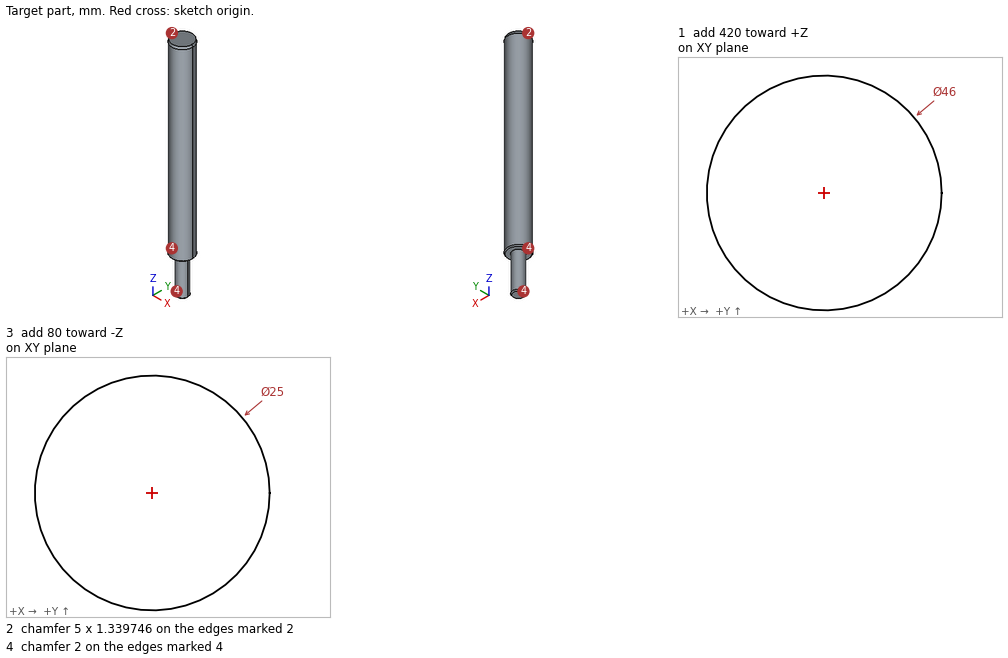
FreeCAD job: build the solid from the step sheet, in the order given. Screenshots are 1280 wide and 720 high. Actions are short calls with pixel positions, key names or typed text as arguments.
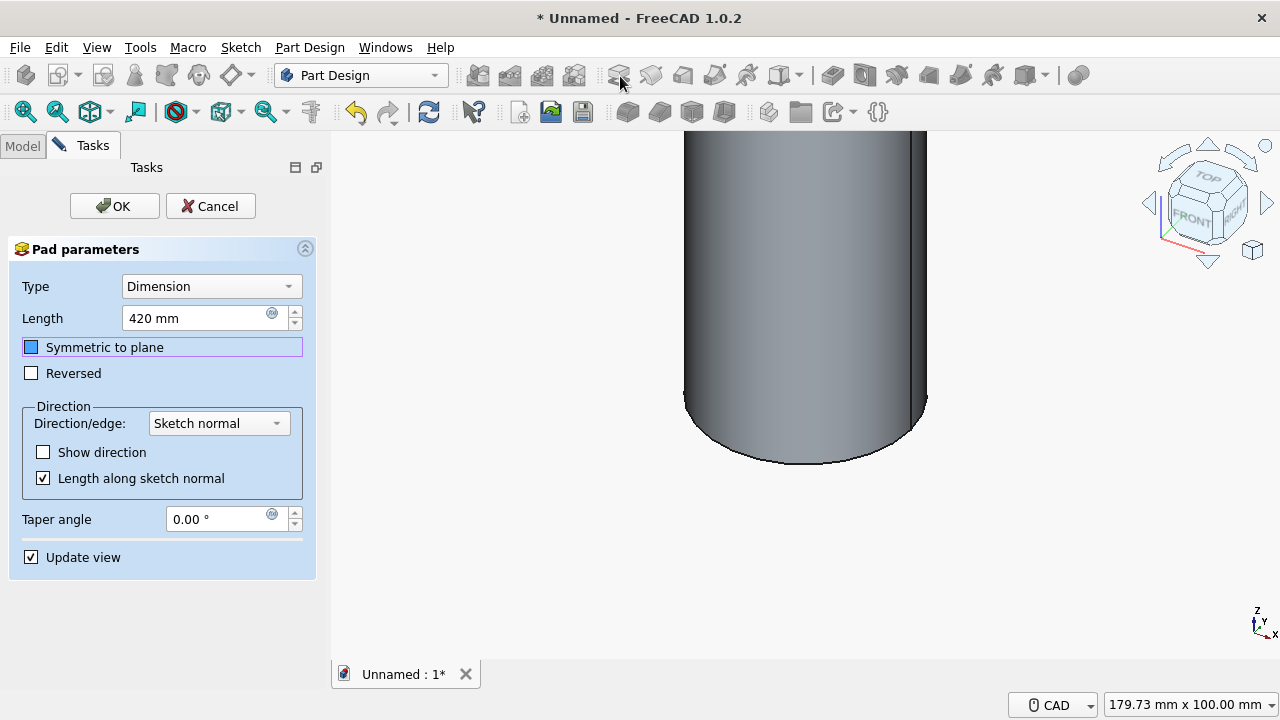
click(115, 206)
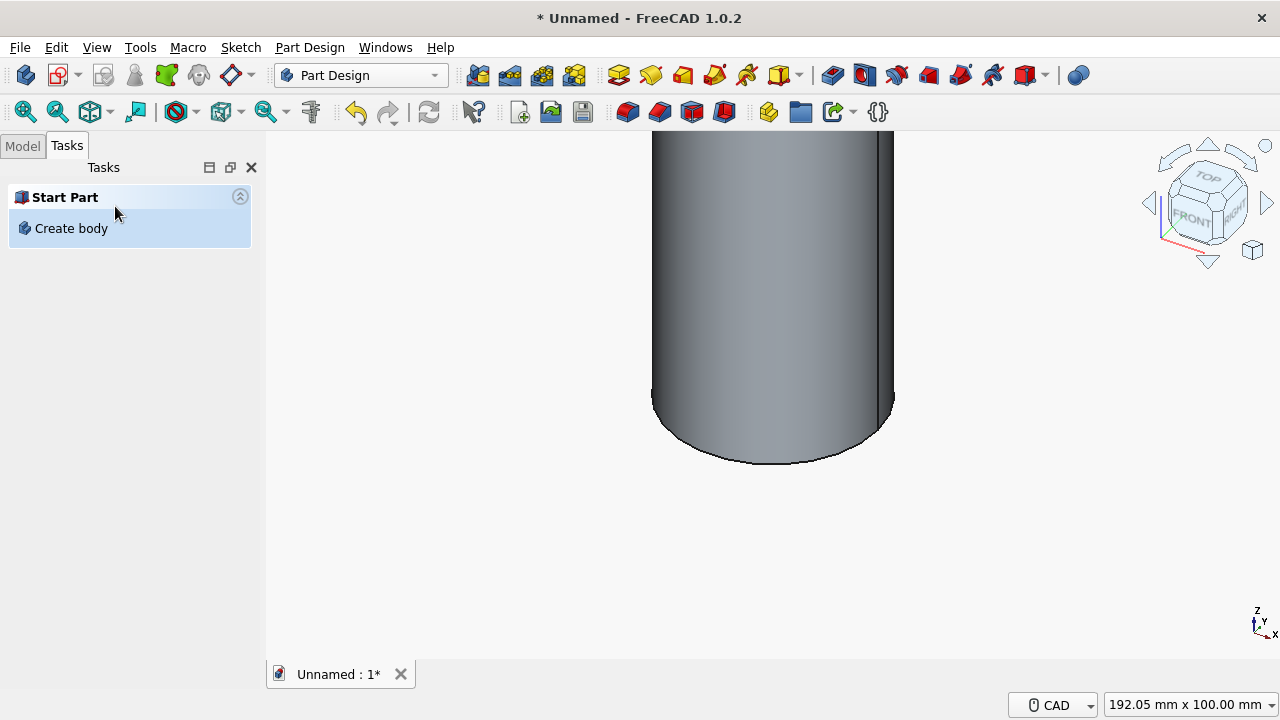
key(v)
key(f)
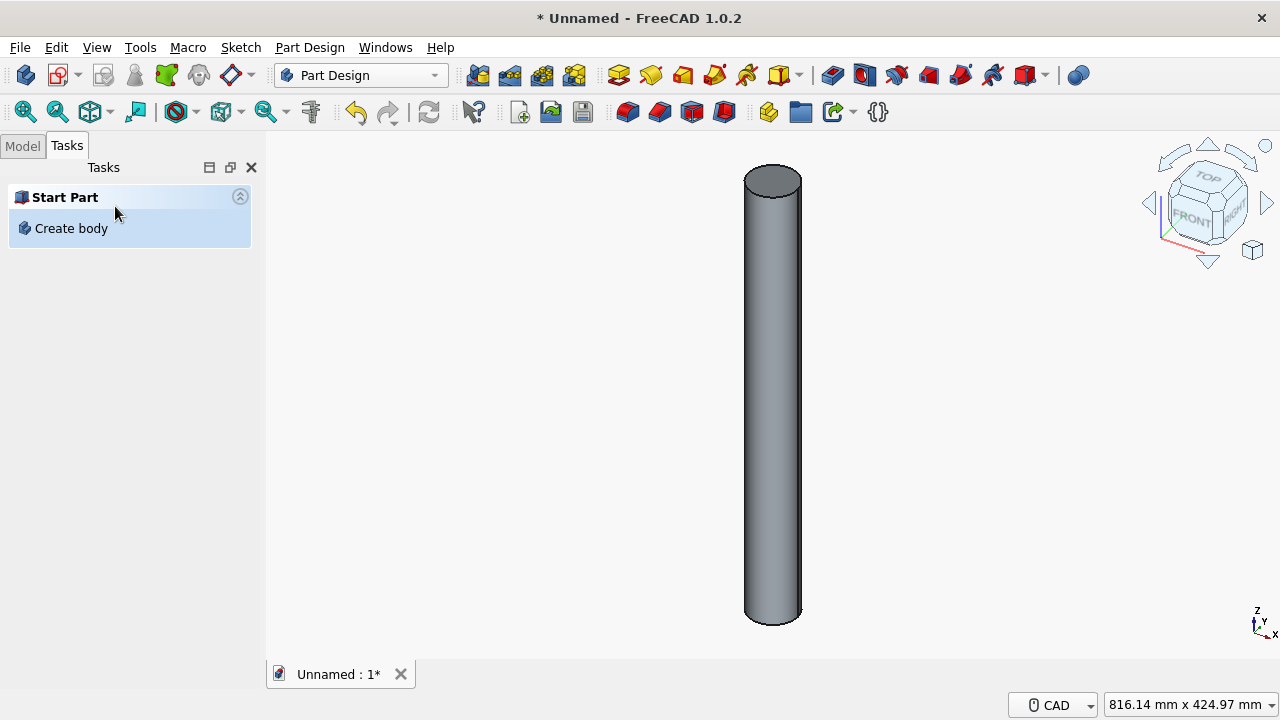
click(761, 165)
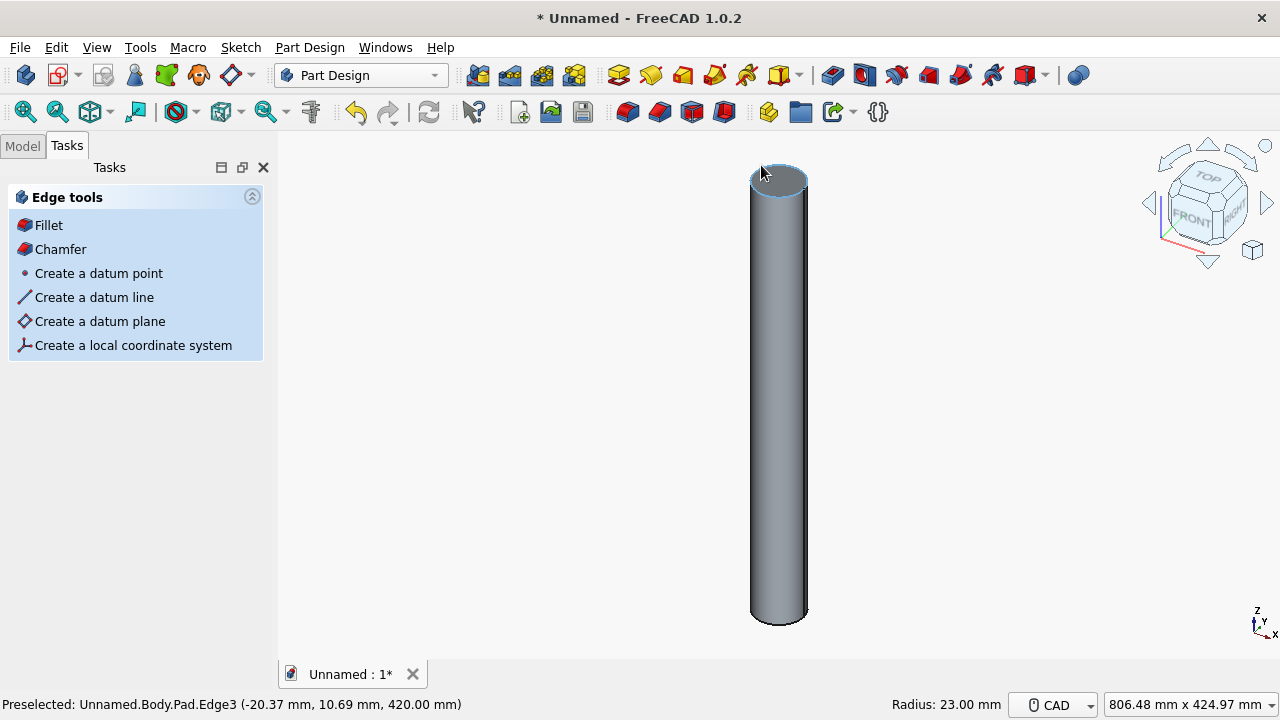
click(660, 112)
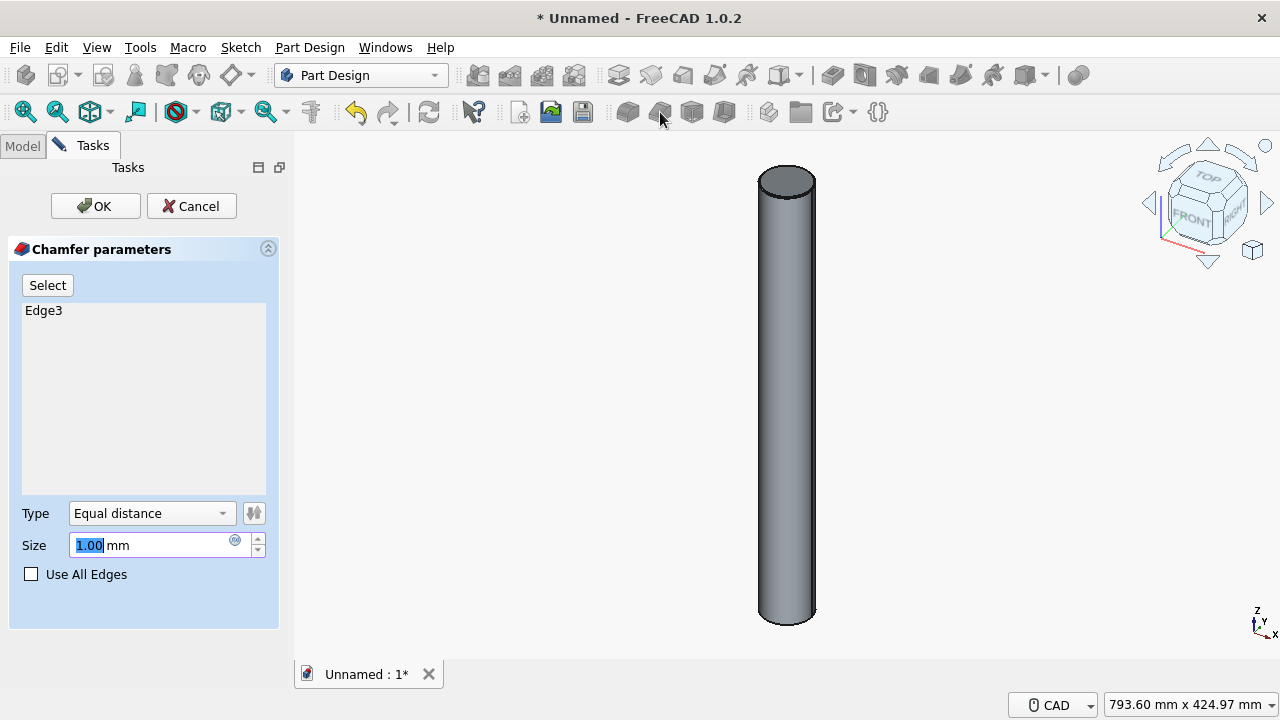
text(5)
key(Tab)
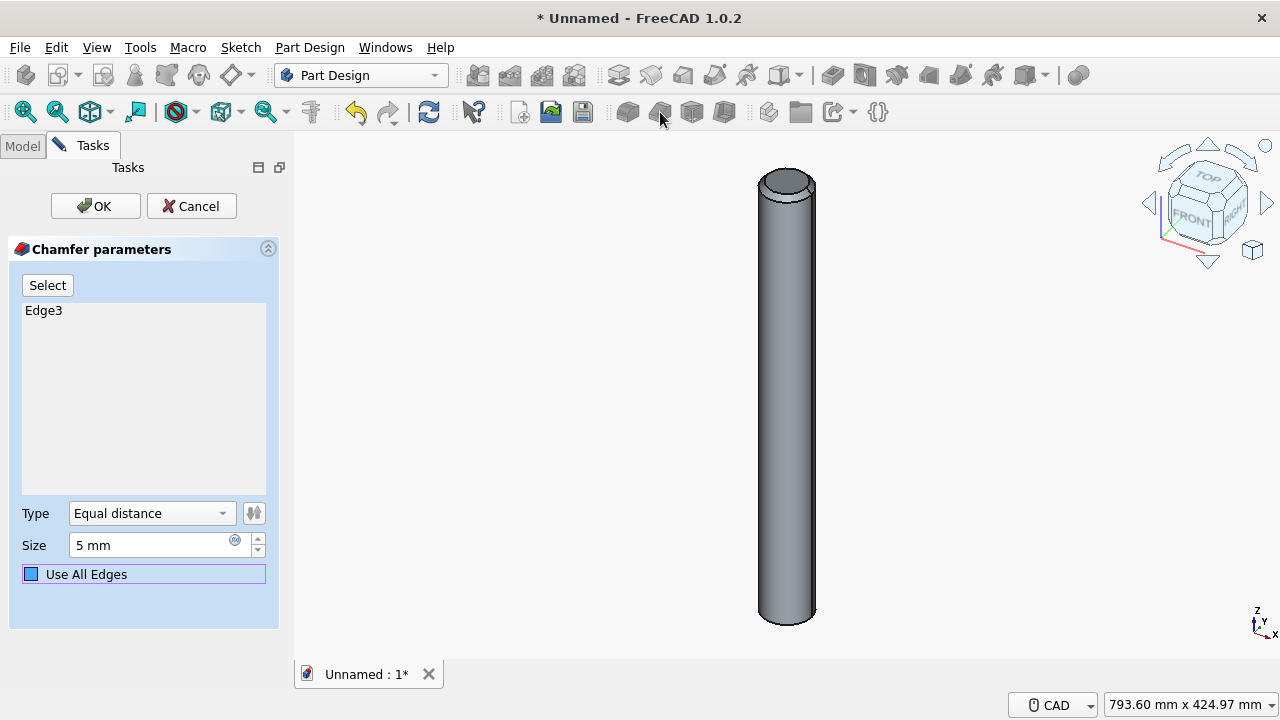
click(153, 514)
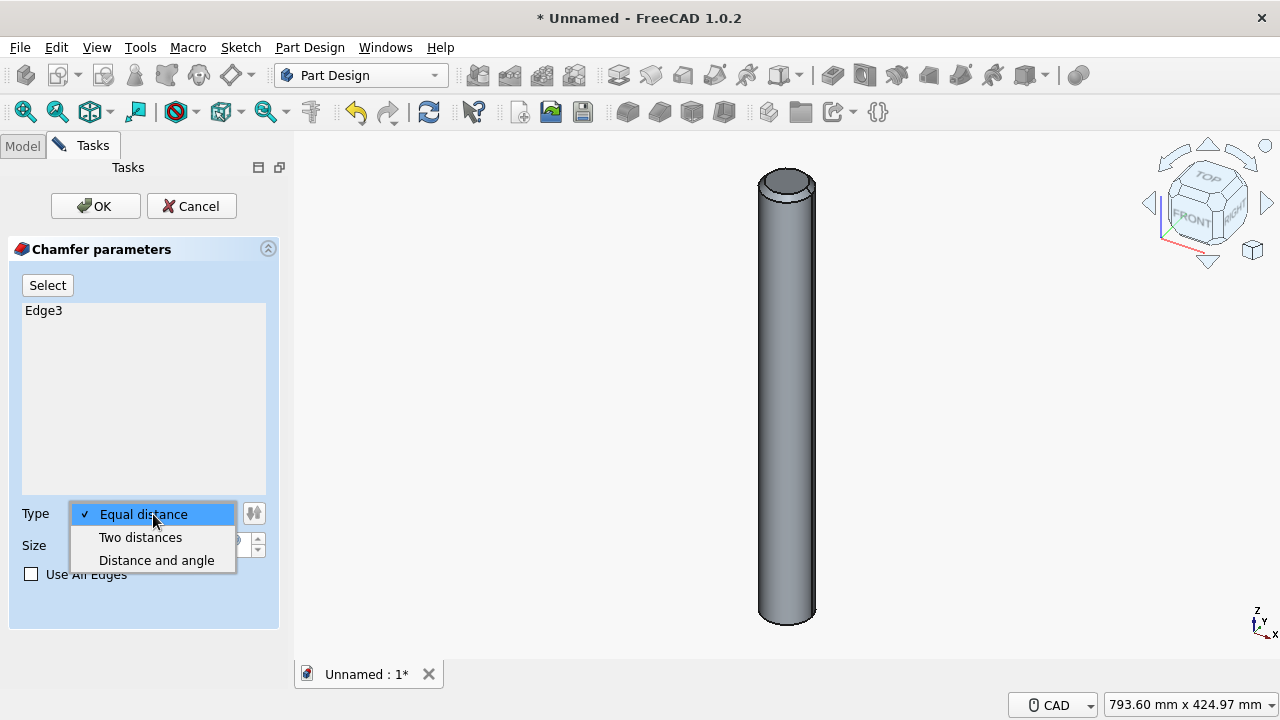
click(152, 538)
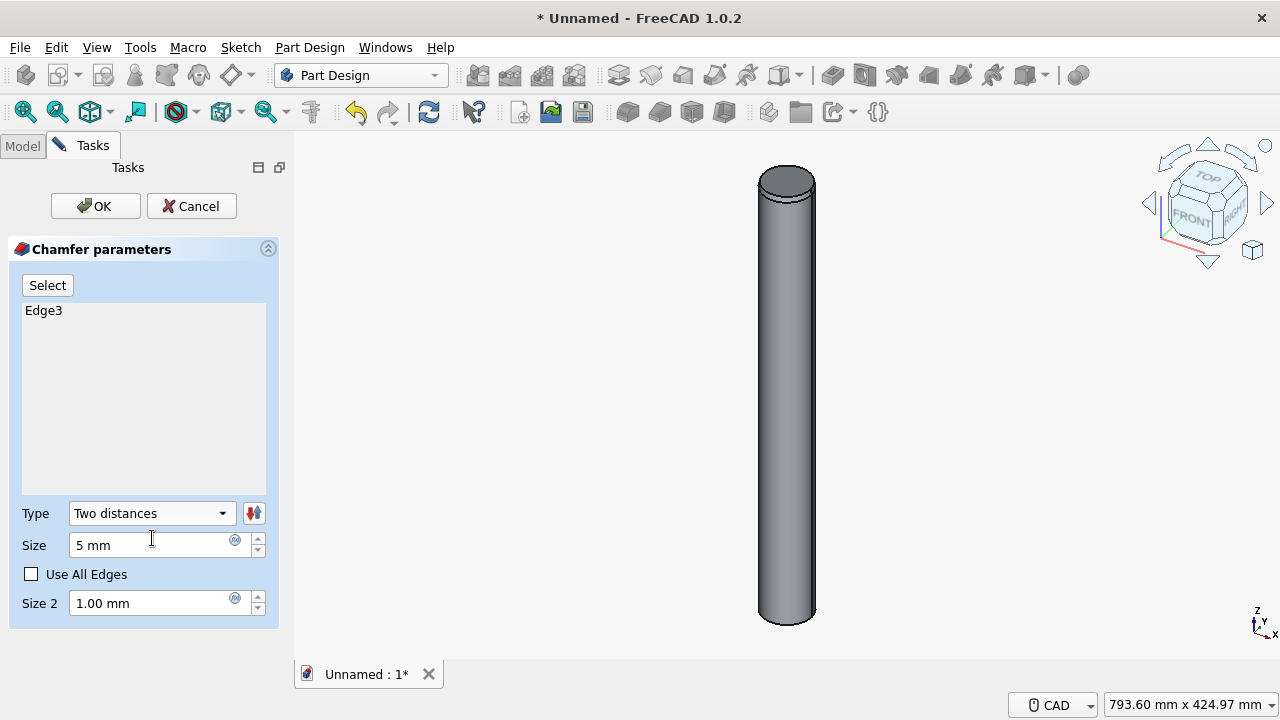
triple_click(160, 603)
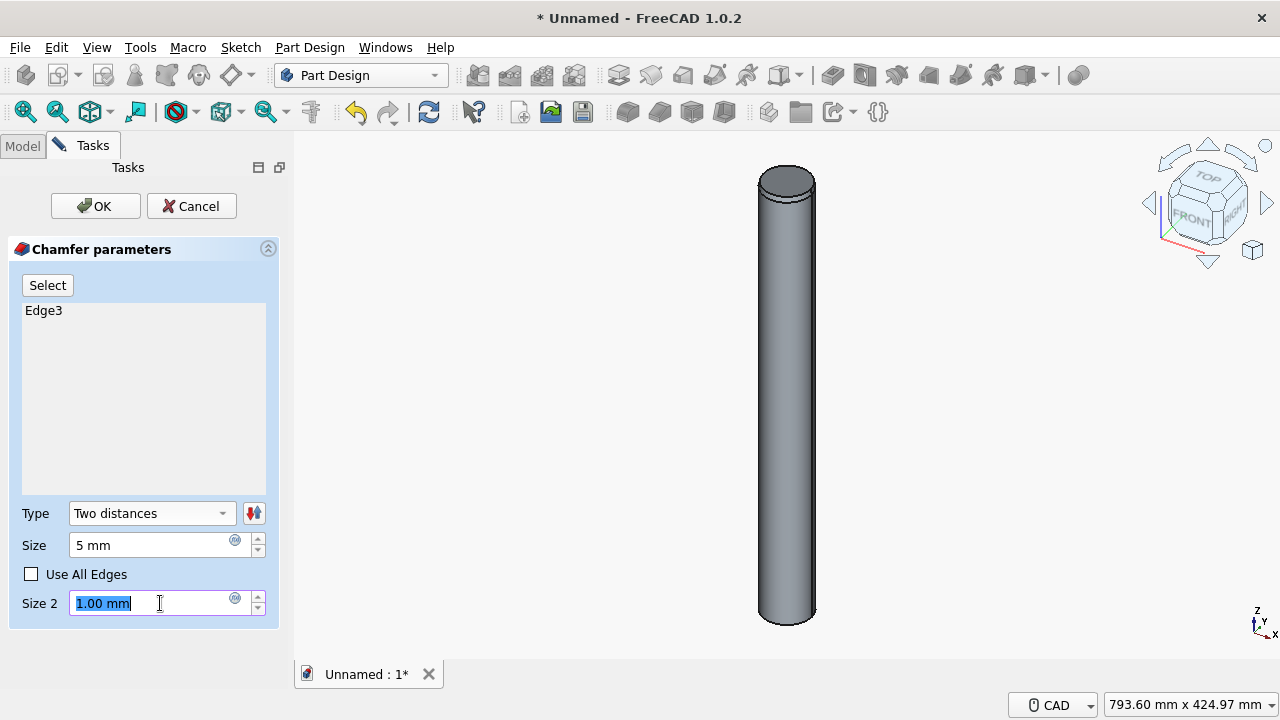
text(1.339746)
key(Tab)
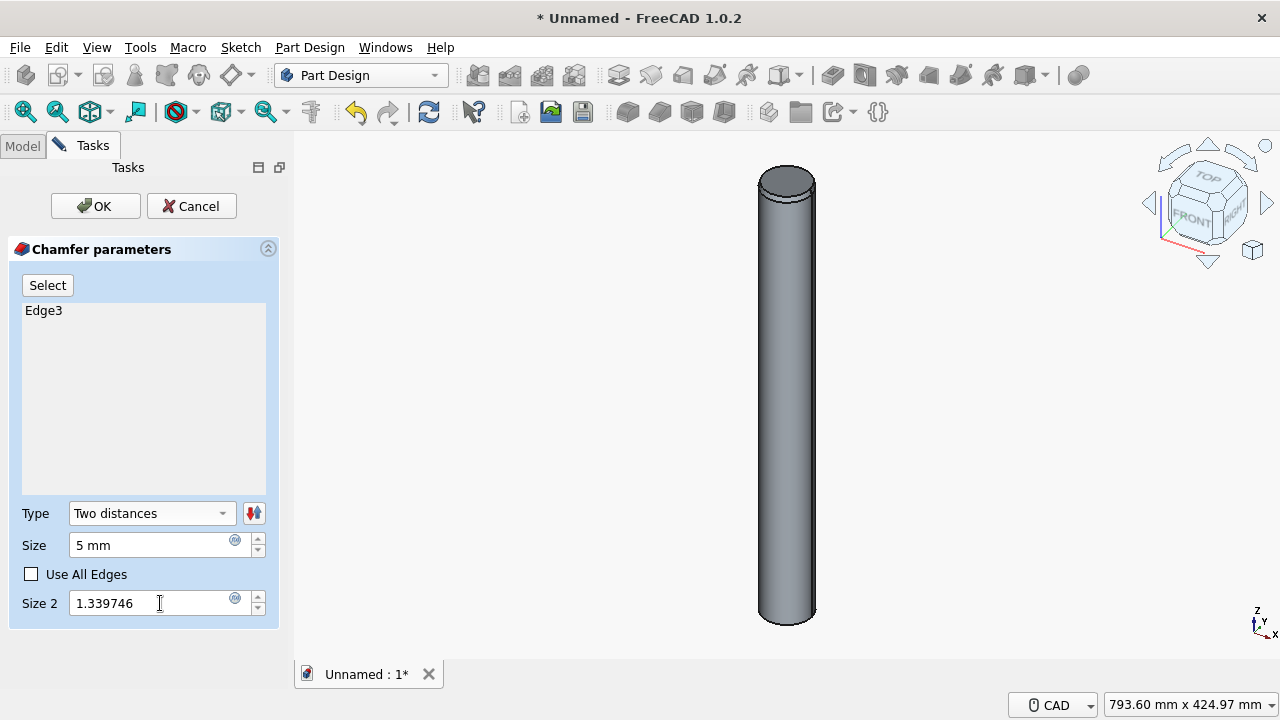
click(96, 206)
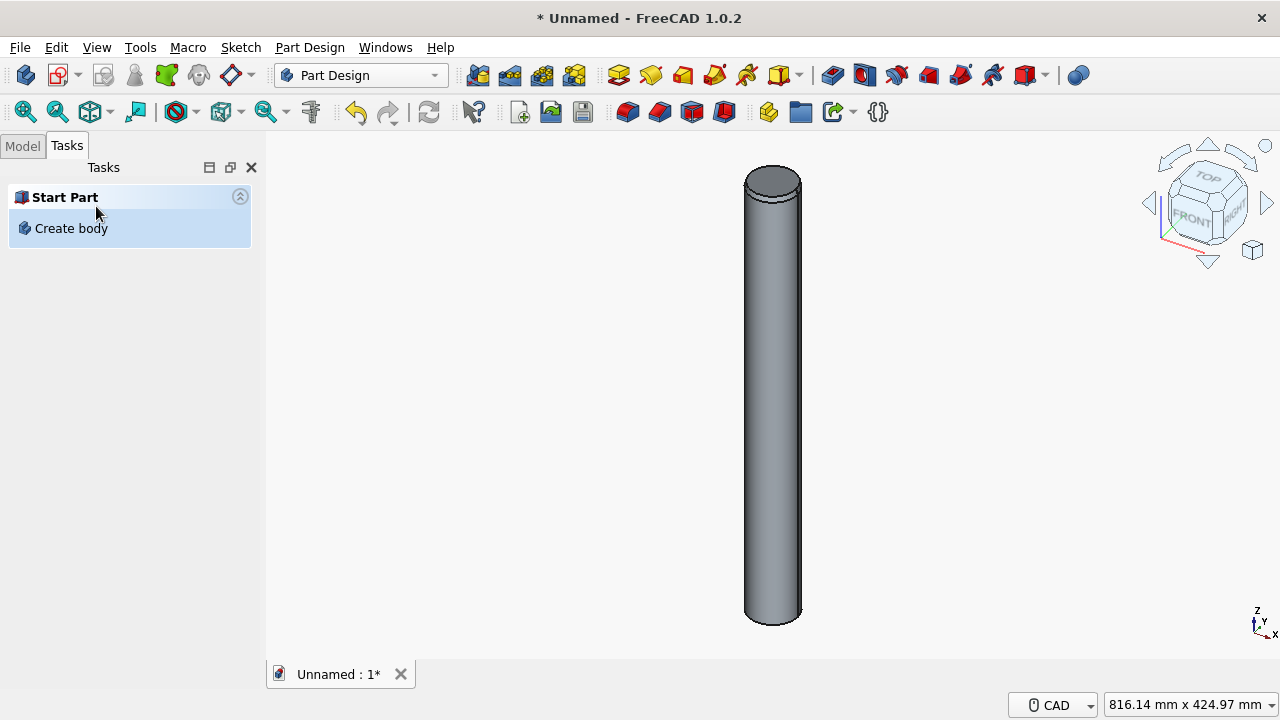
click(58, 76)